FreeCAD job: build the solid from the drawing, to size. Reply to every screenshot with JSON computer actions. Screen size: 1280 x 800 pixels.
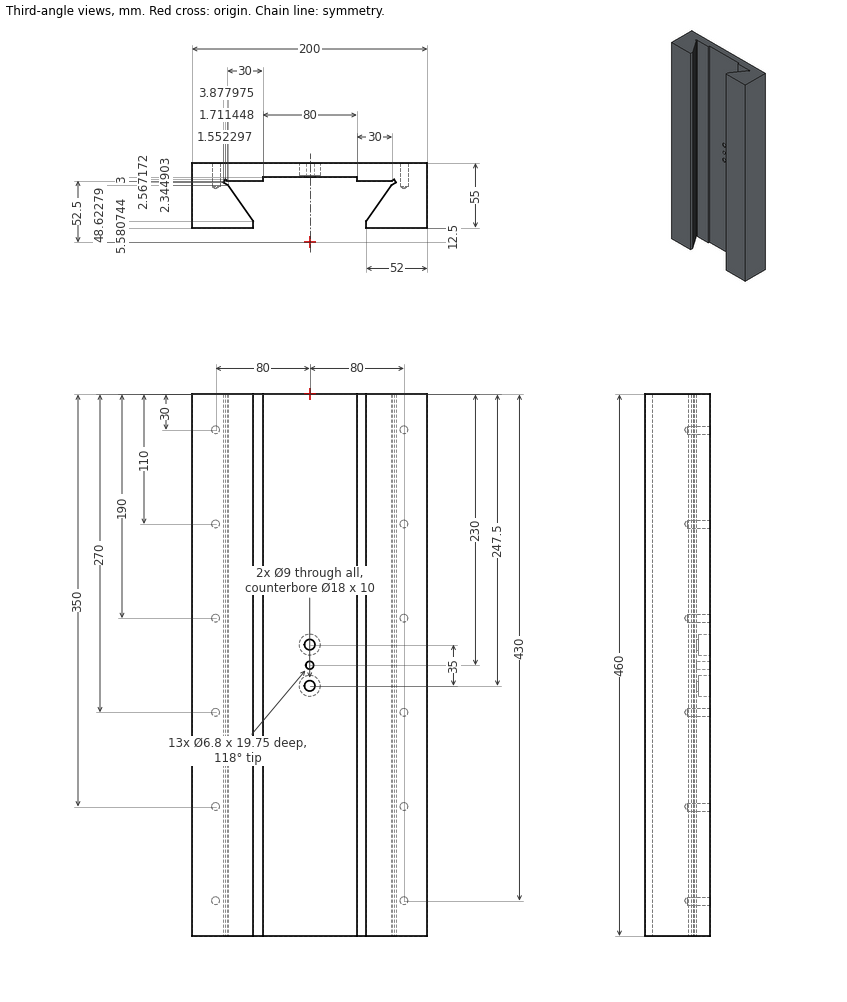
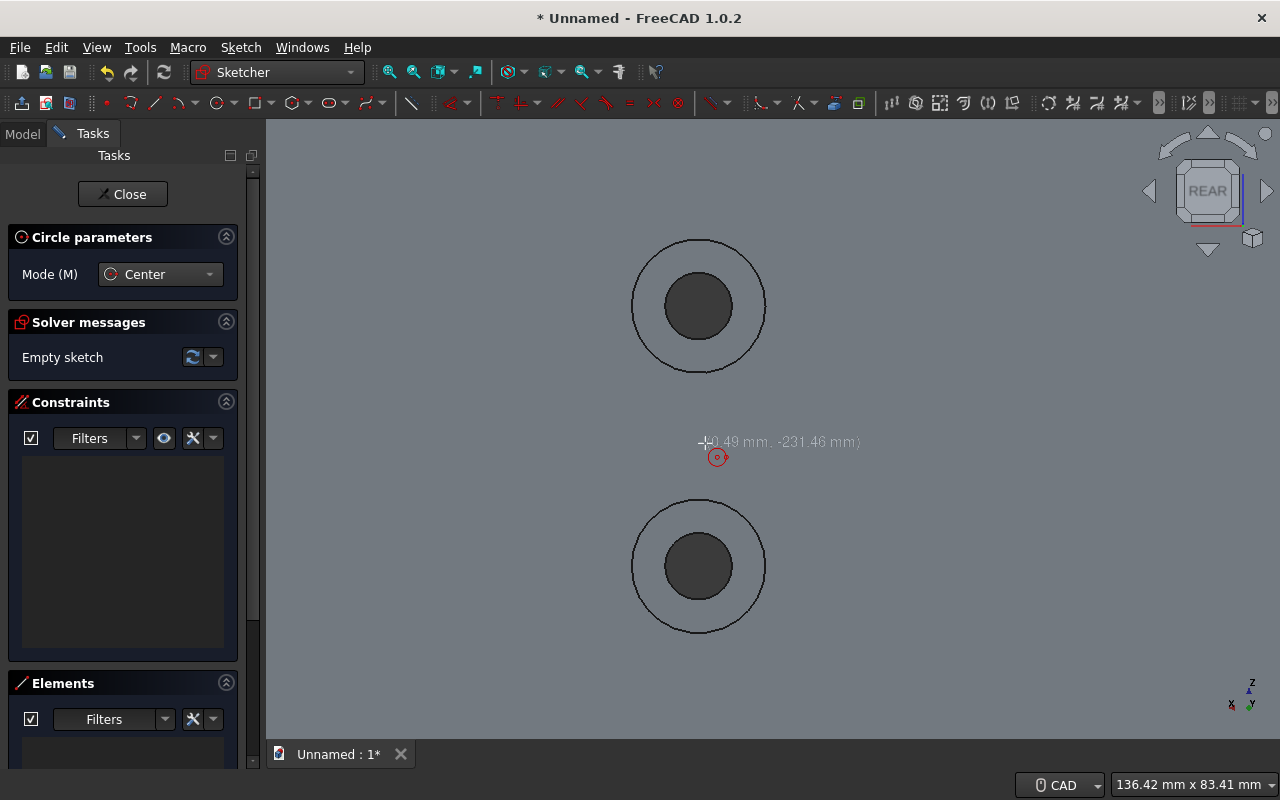
{"action": "scroll", "coordinate": [705, 443], "scroll_direction": "down", "scroll_amount": 10}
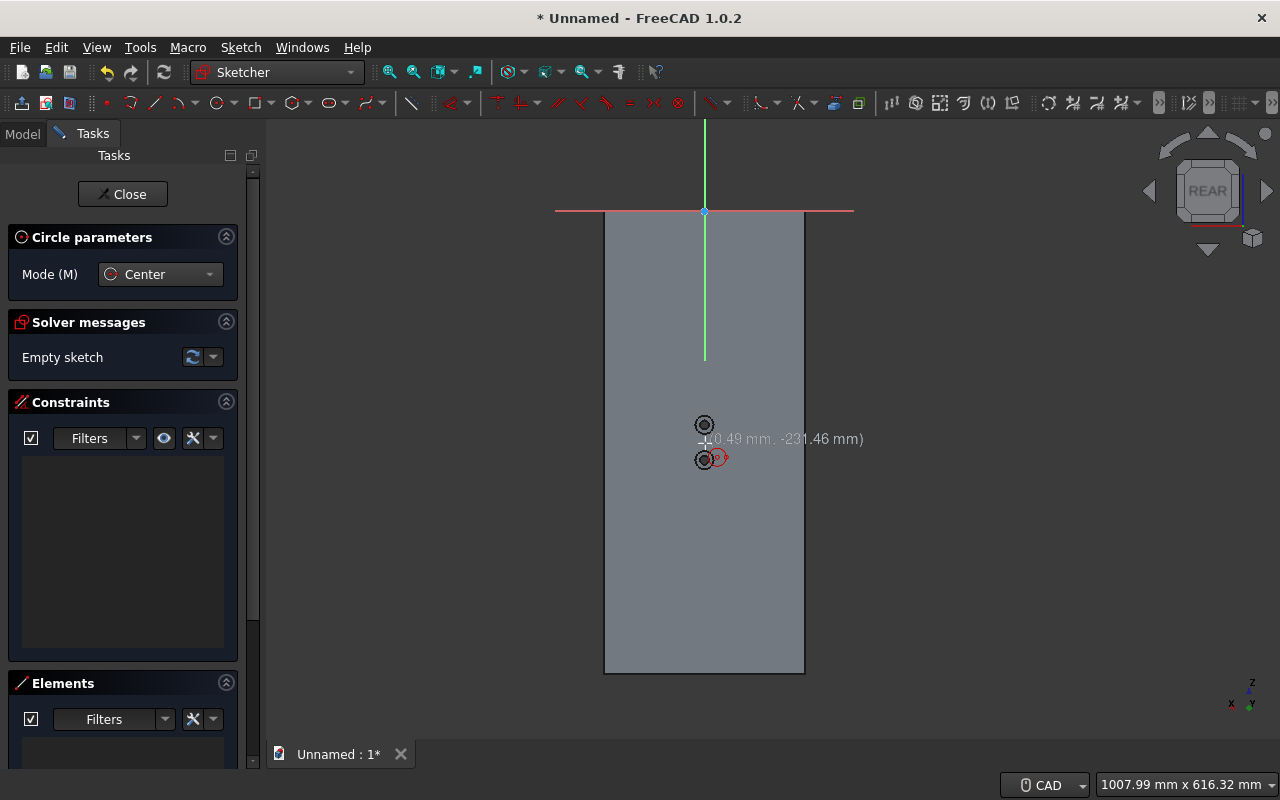
{"action": "left_click", "coordinate": [705, 443]}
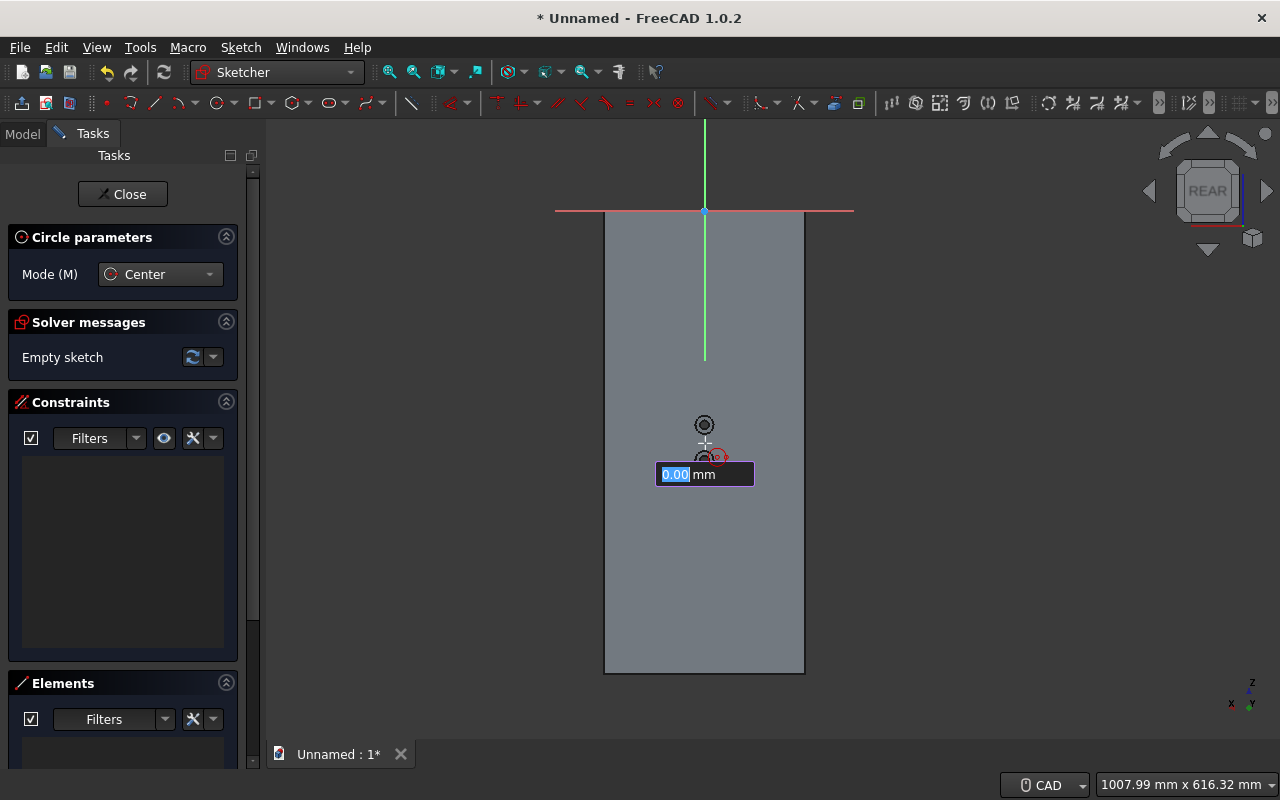
{"action": "scroll", "coordinate": [708, 441], "scroll_direction": "up", "scroll_amount": 8}
{"action": "mouse_move", "coordinate": [705, 441]}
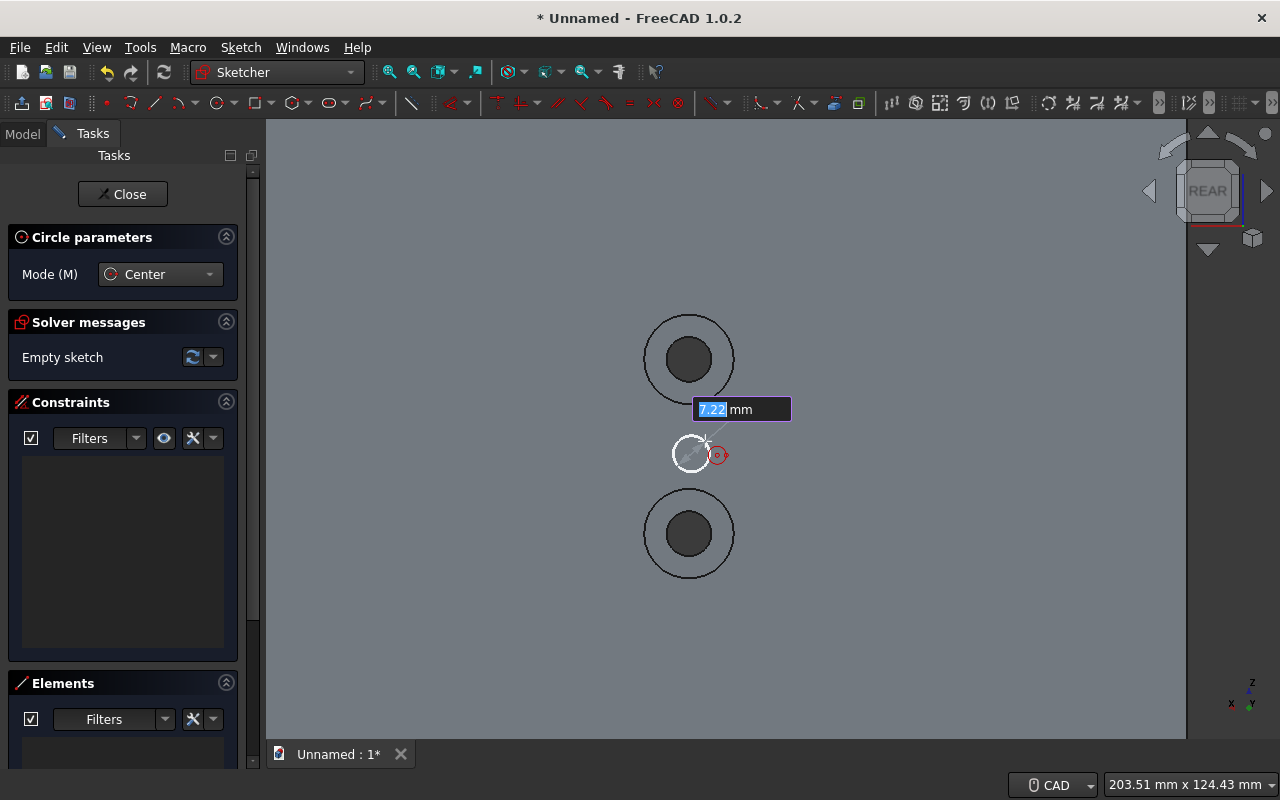
{"action": "type", "text": "6.8"}
{"action": "key", "text": "Return"}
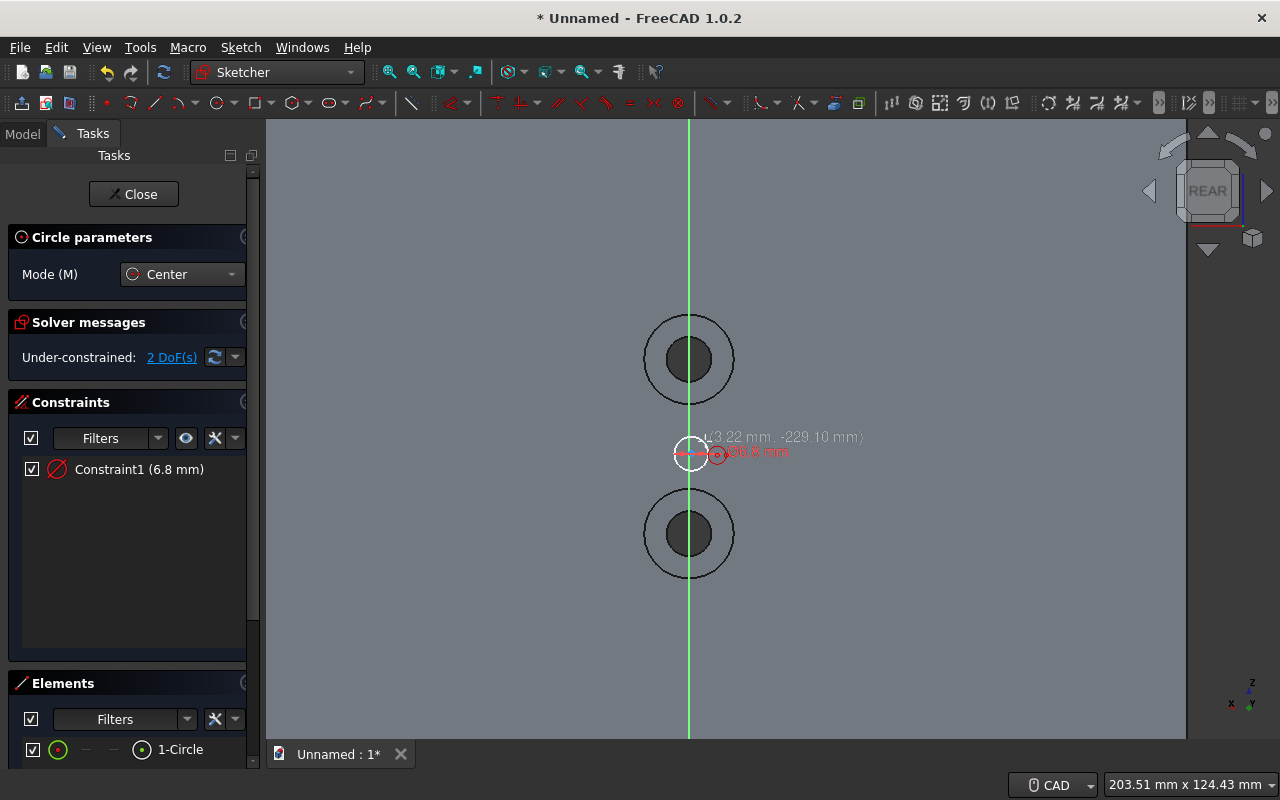
{"action": "scroll", "coordinate": [708, 441], "scroll_direction": "down", "scroll_amount": 8}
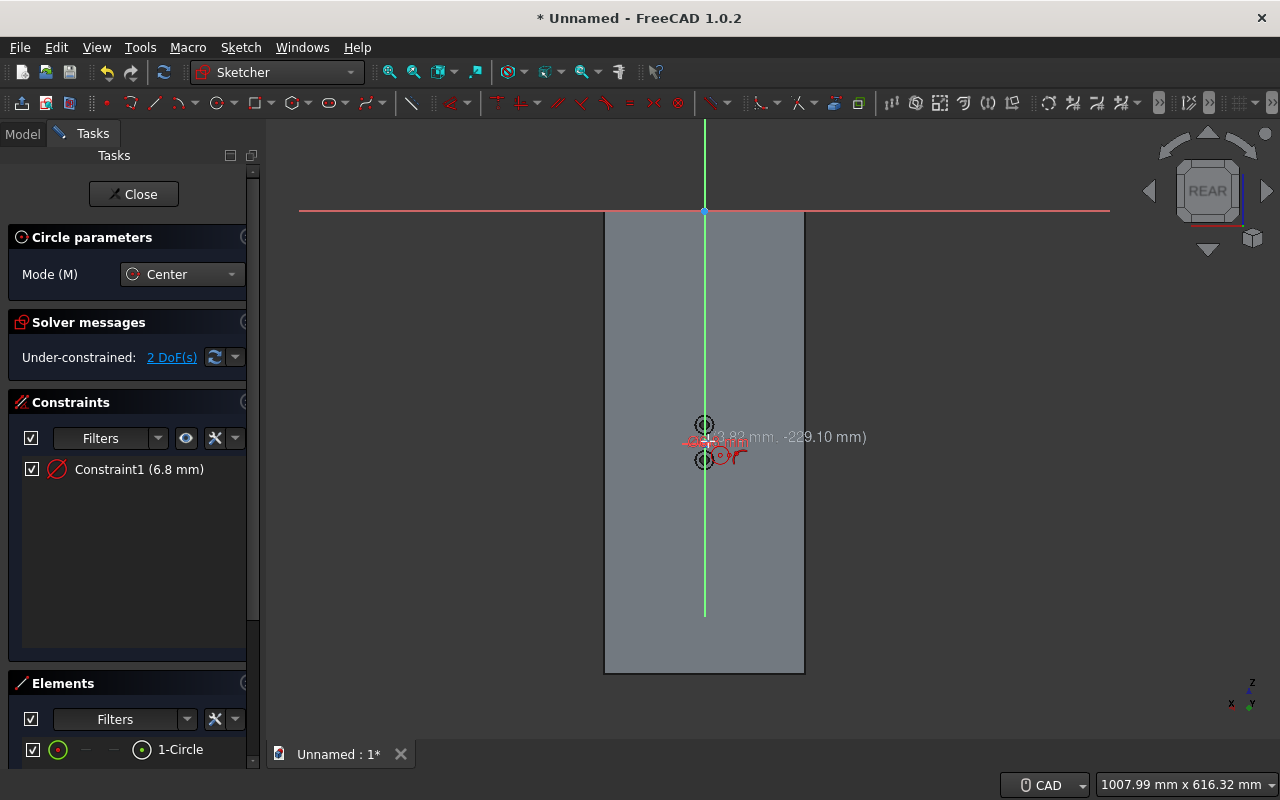
{"action": "scroll", "coordinate": [624, 644], "scroll_direction": "up", "scroll_amount": 10}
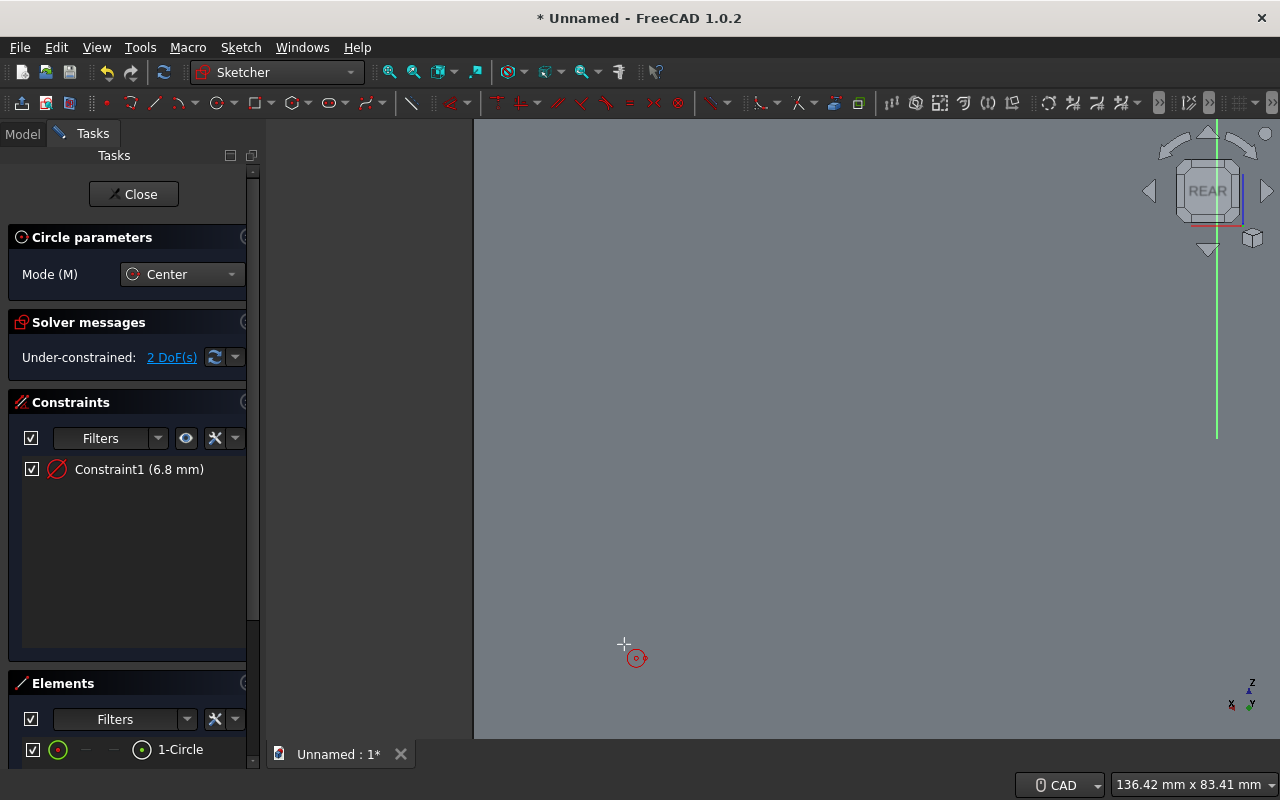
{"action": "scroll", "coordinate": [624, 645], "scroll_direction": "down", "scroll_amount": 10}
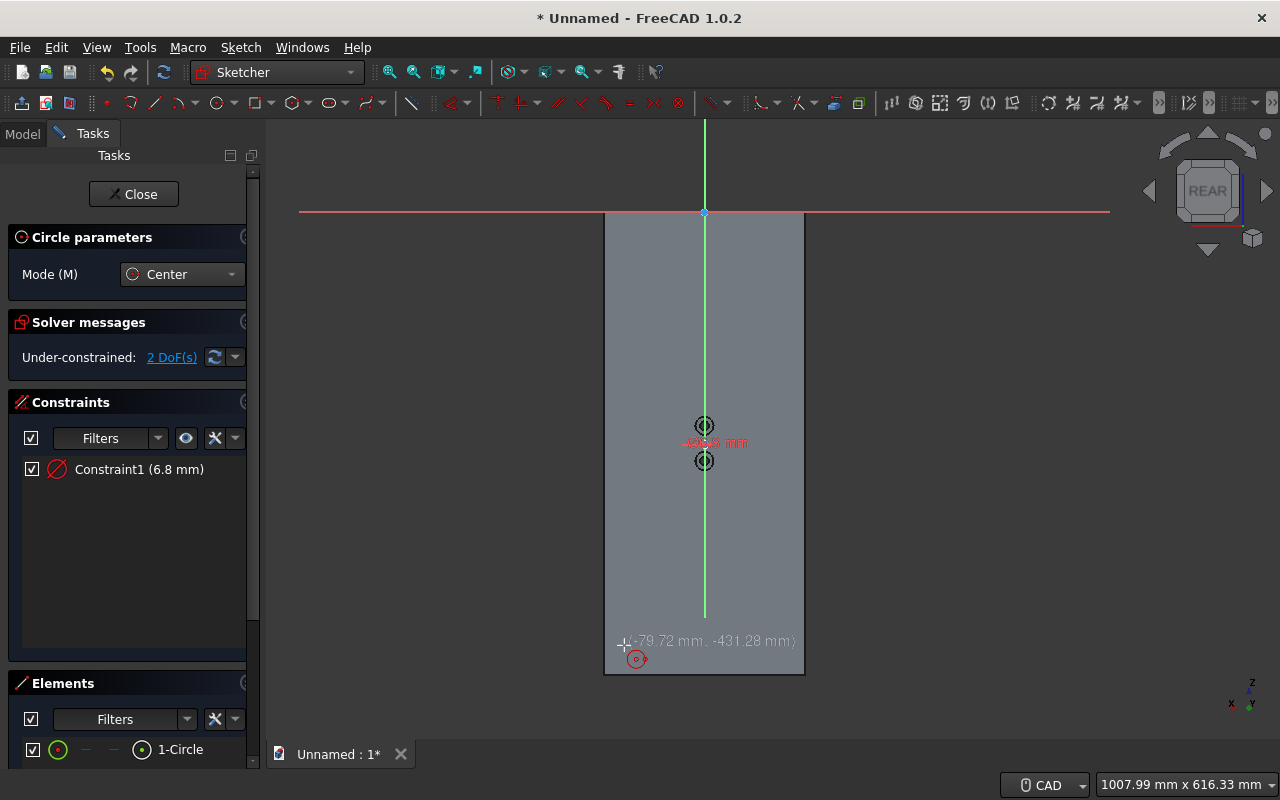
{"action": "left_click", "coordinate": [624, 645]}
{"action": "mouse_move", "coordinate": [626, 642]}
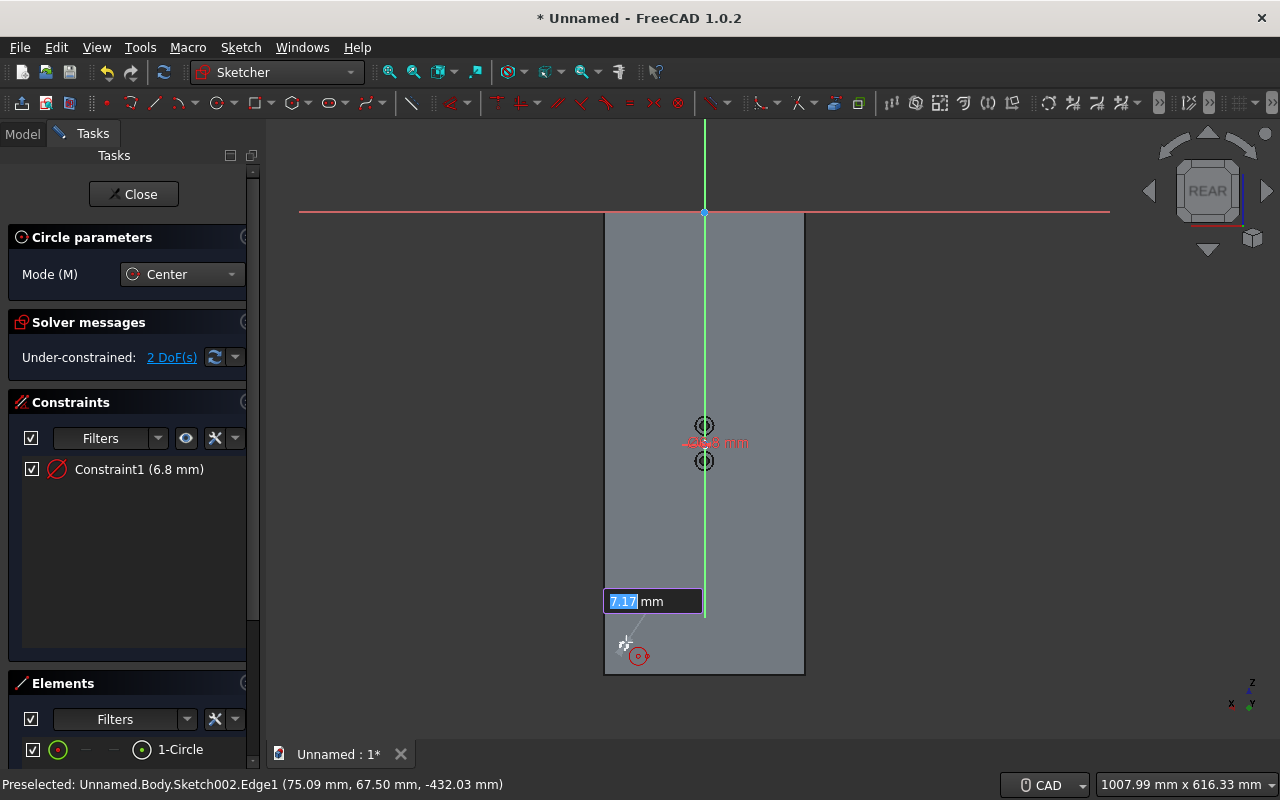
{"action": "type", "text": "6.8"}
{"action": "key", "text": "Return"}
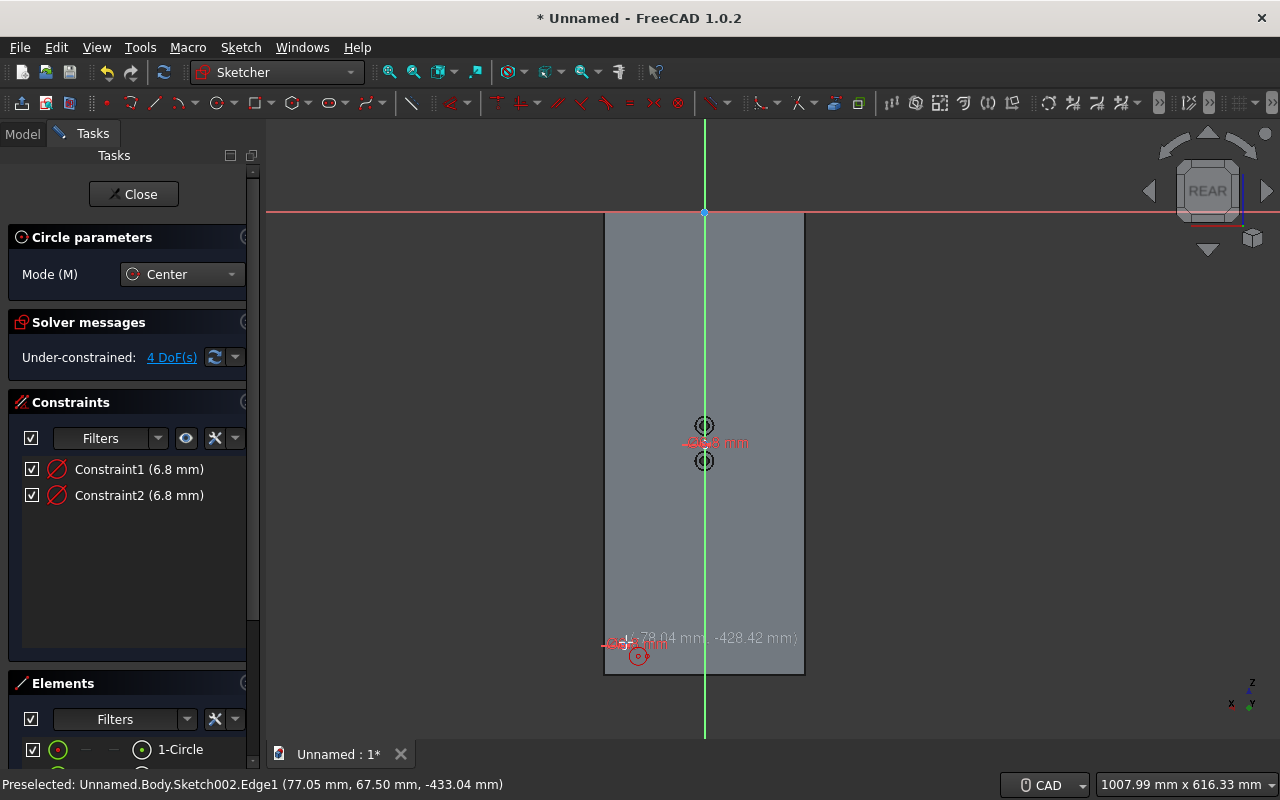
{"action": "scroll", "coordinate": [785, 242], "scroll_direction": "up", "scroll_amount": 10}